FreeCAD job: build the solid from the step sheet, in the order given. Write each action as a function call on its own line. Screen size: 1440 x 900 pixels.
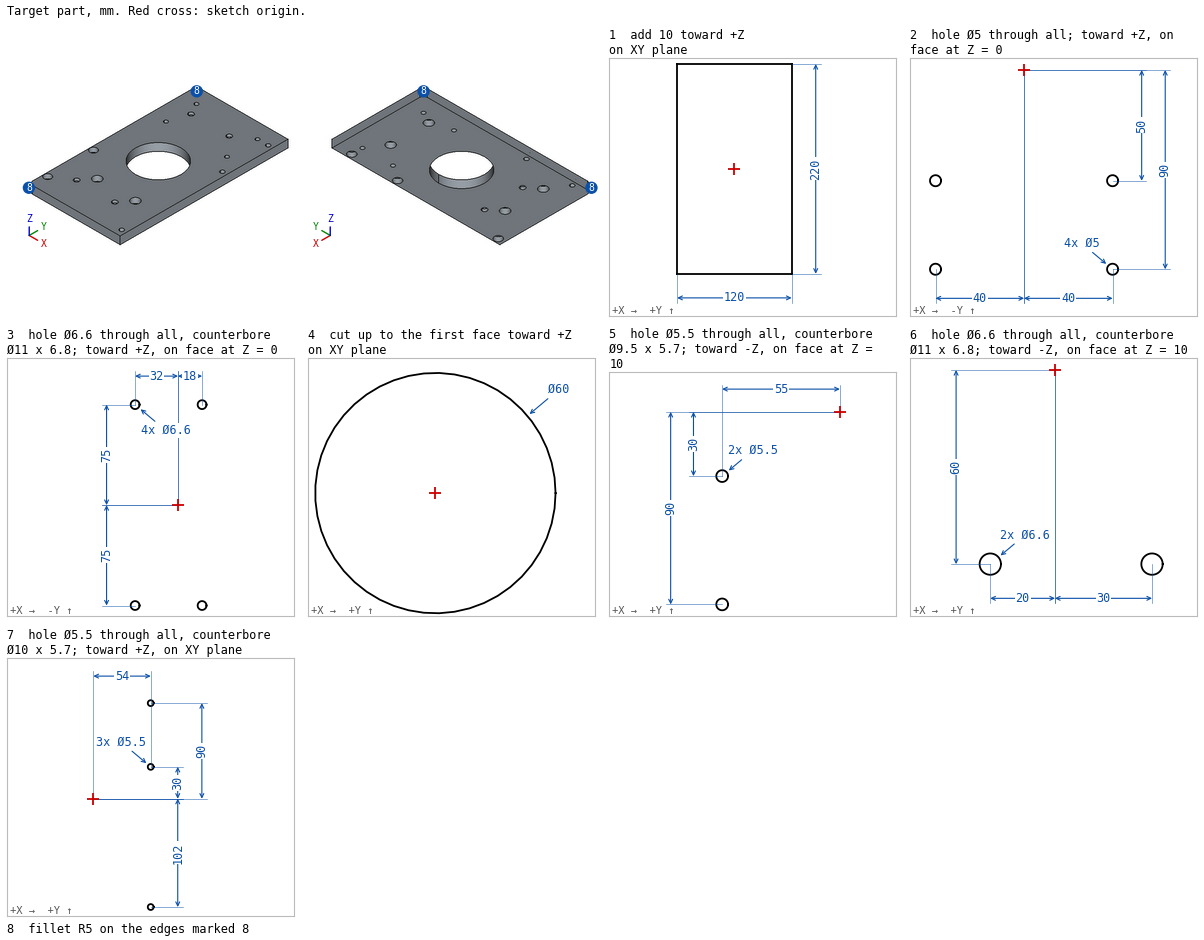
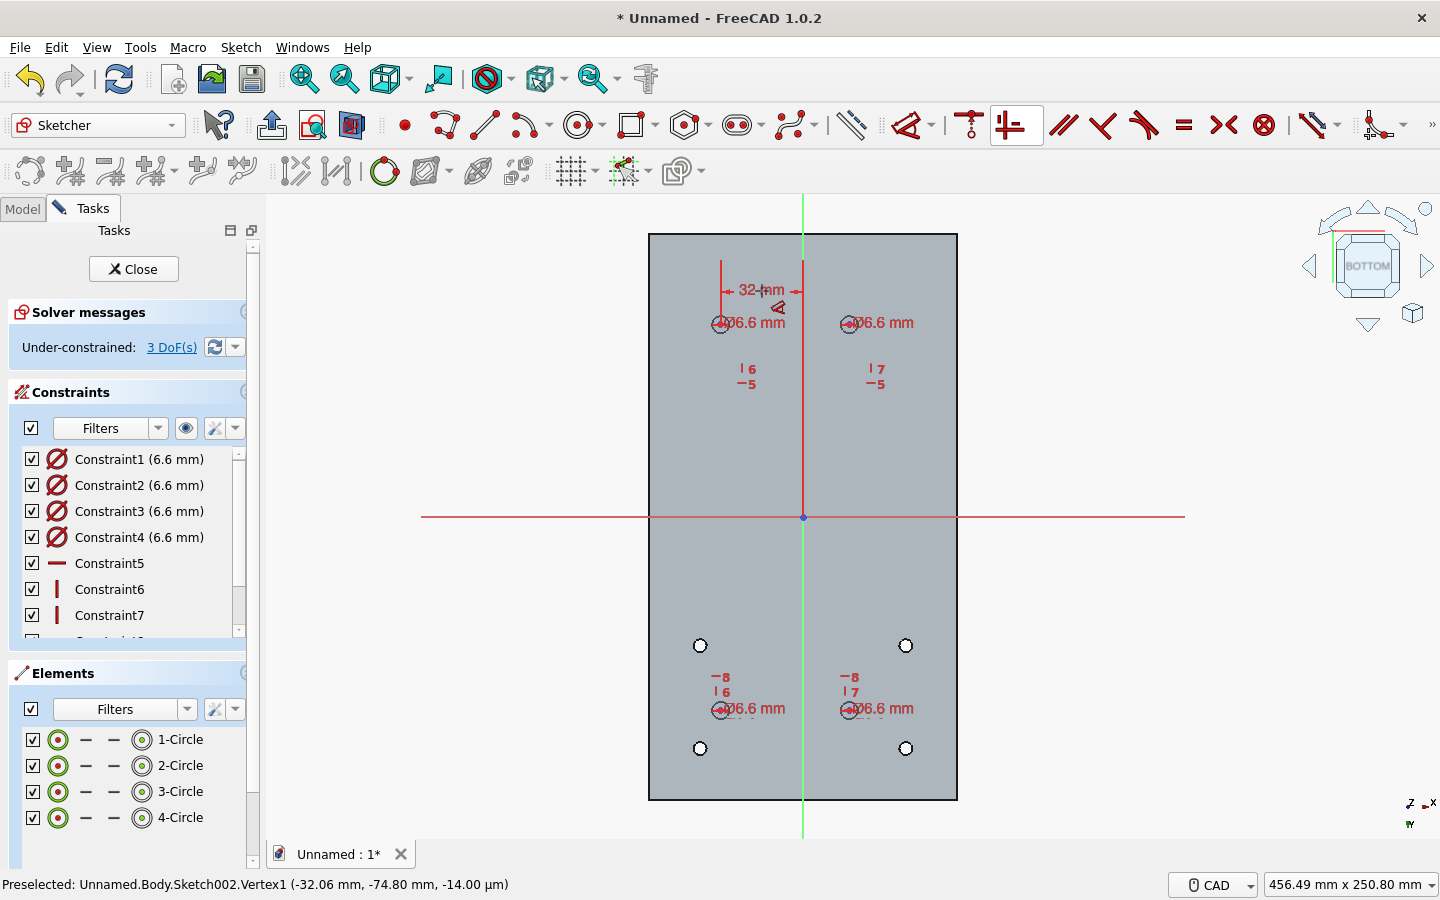
click(721, 325)
click(687, 421)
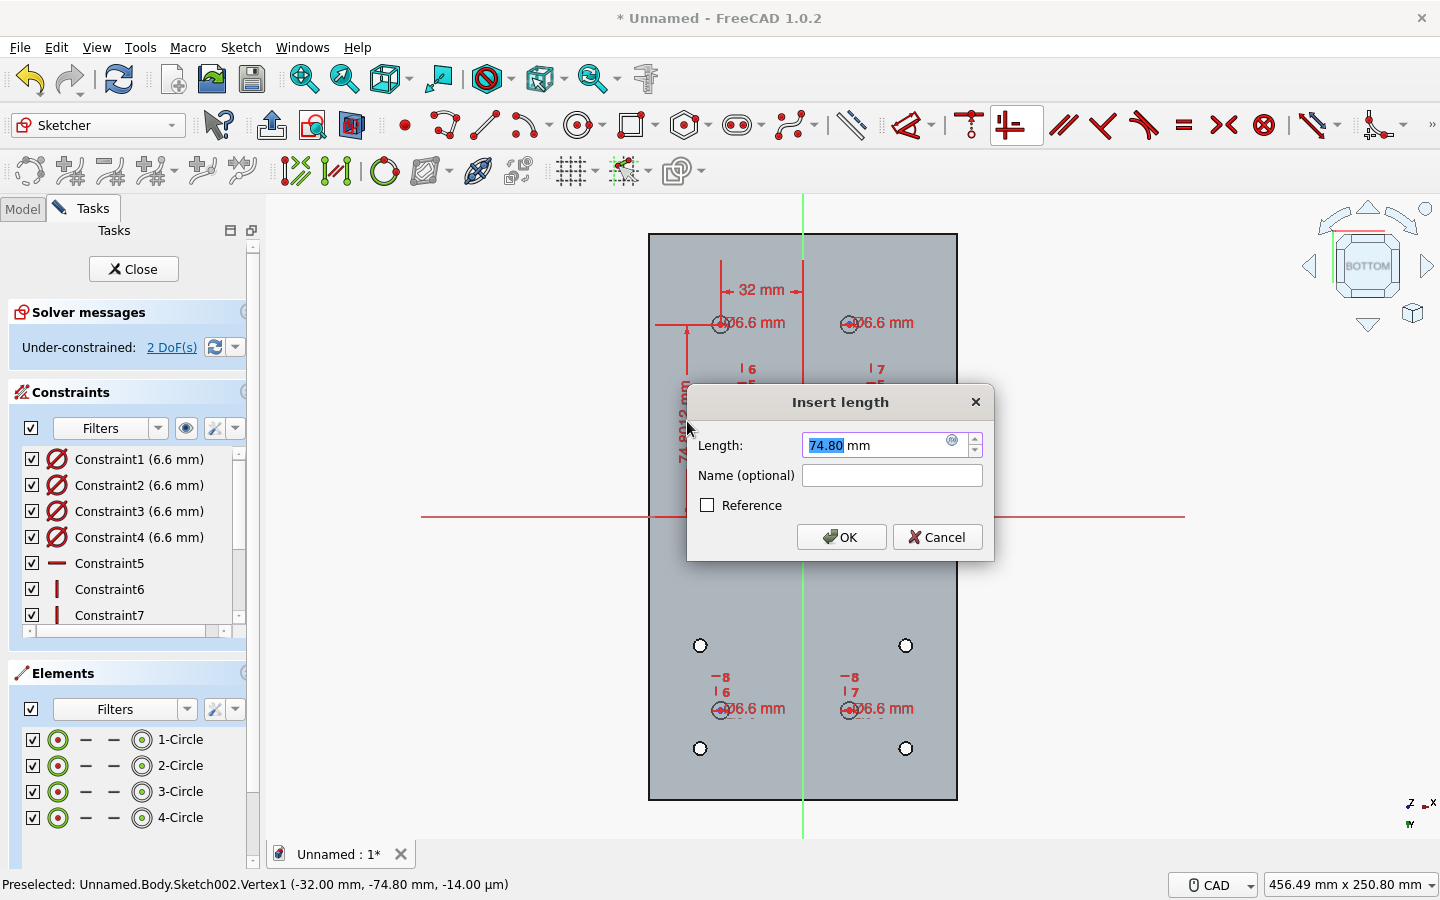
text(75)
key(Return)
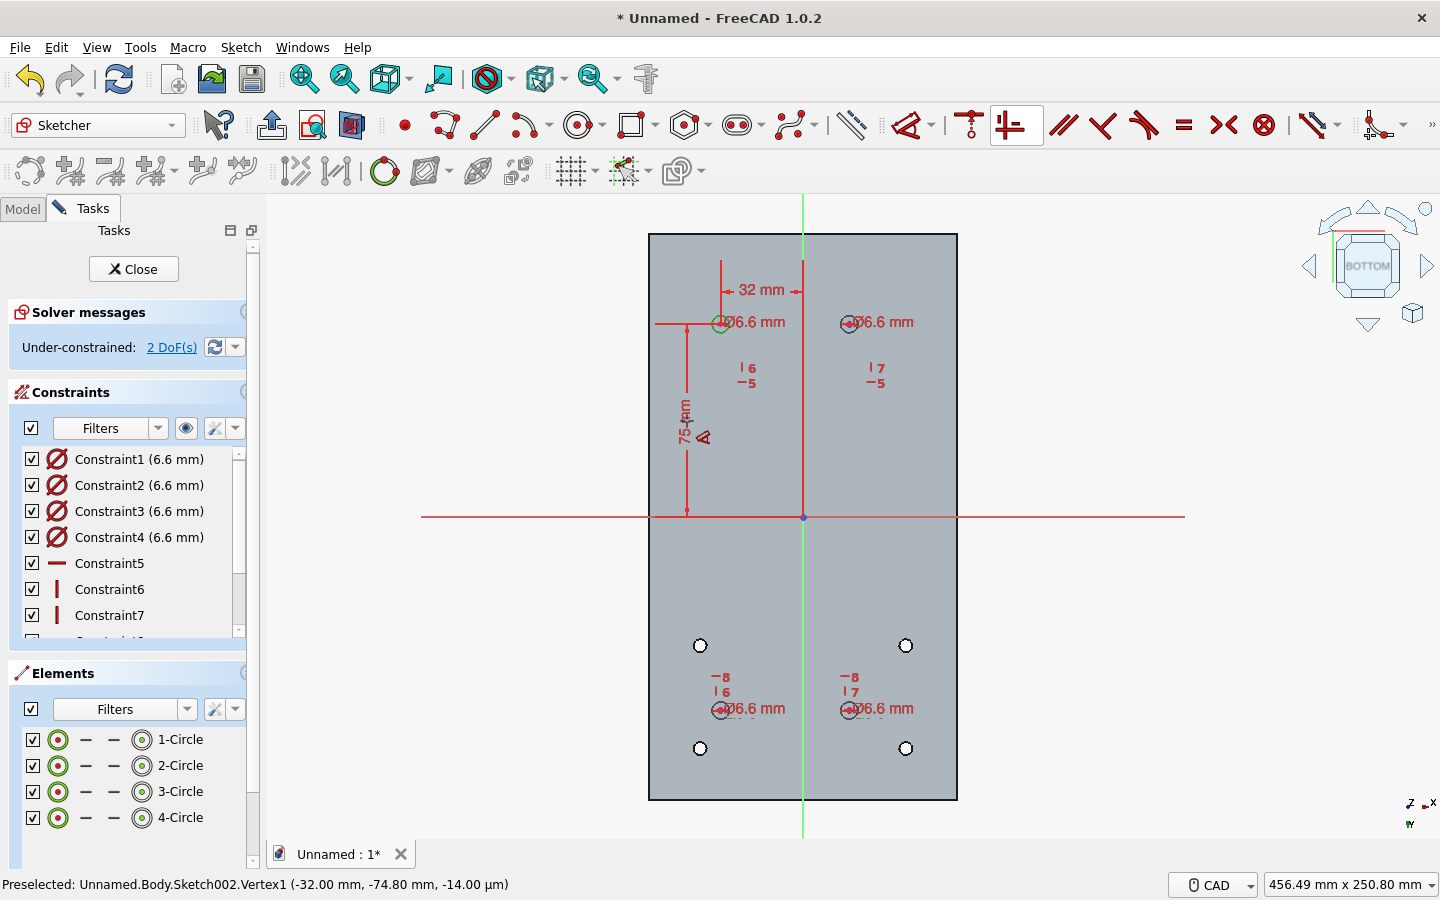
click(849, 324)
click(837, 290)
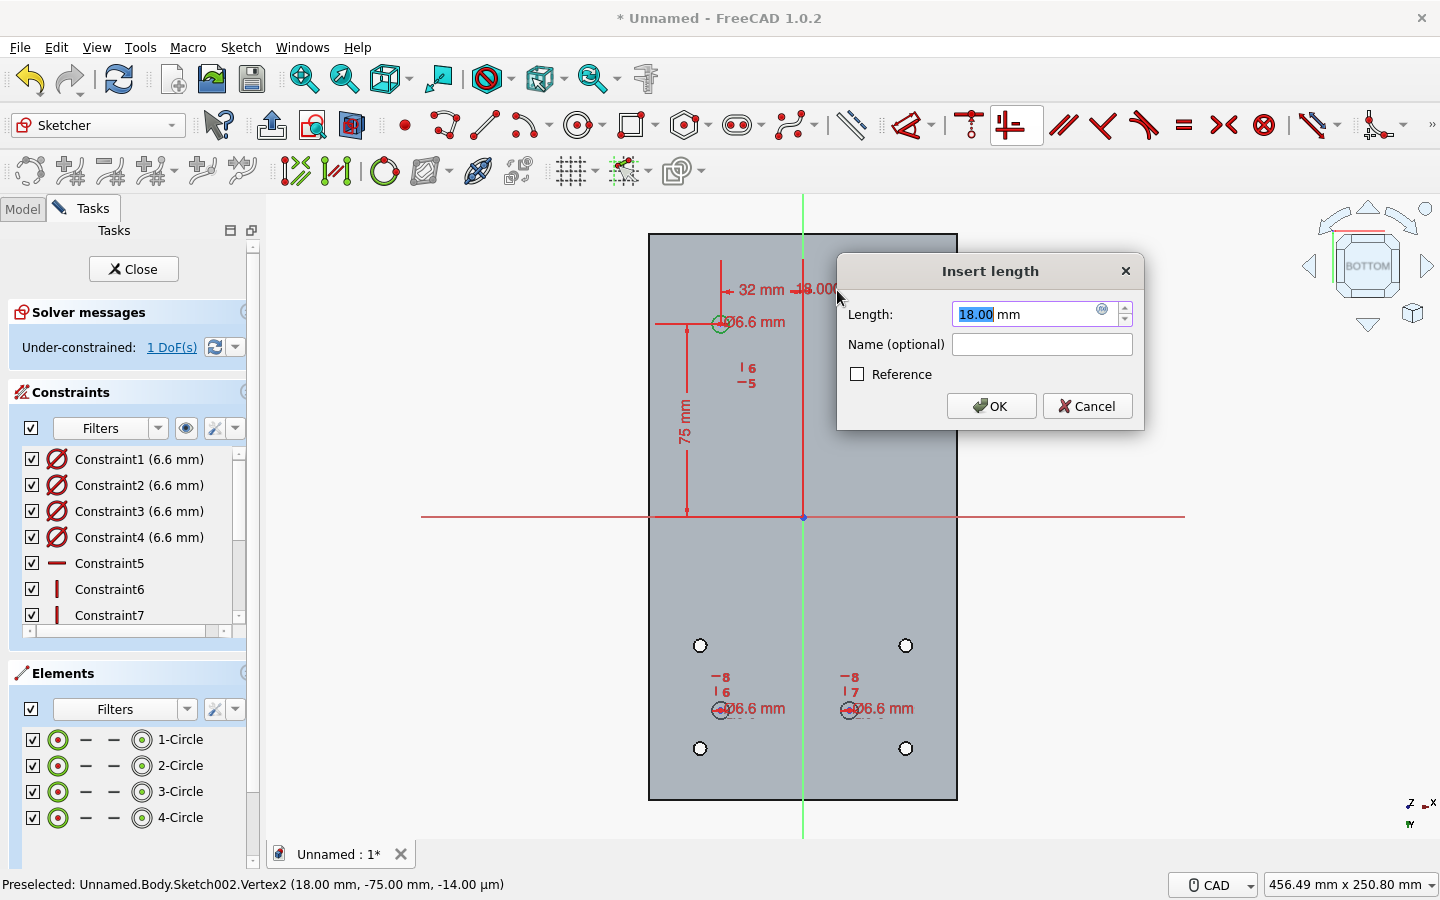
text(18)
key(Return)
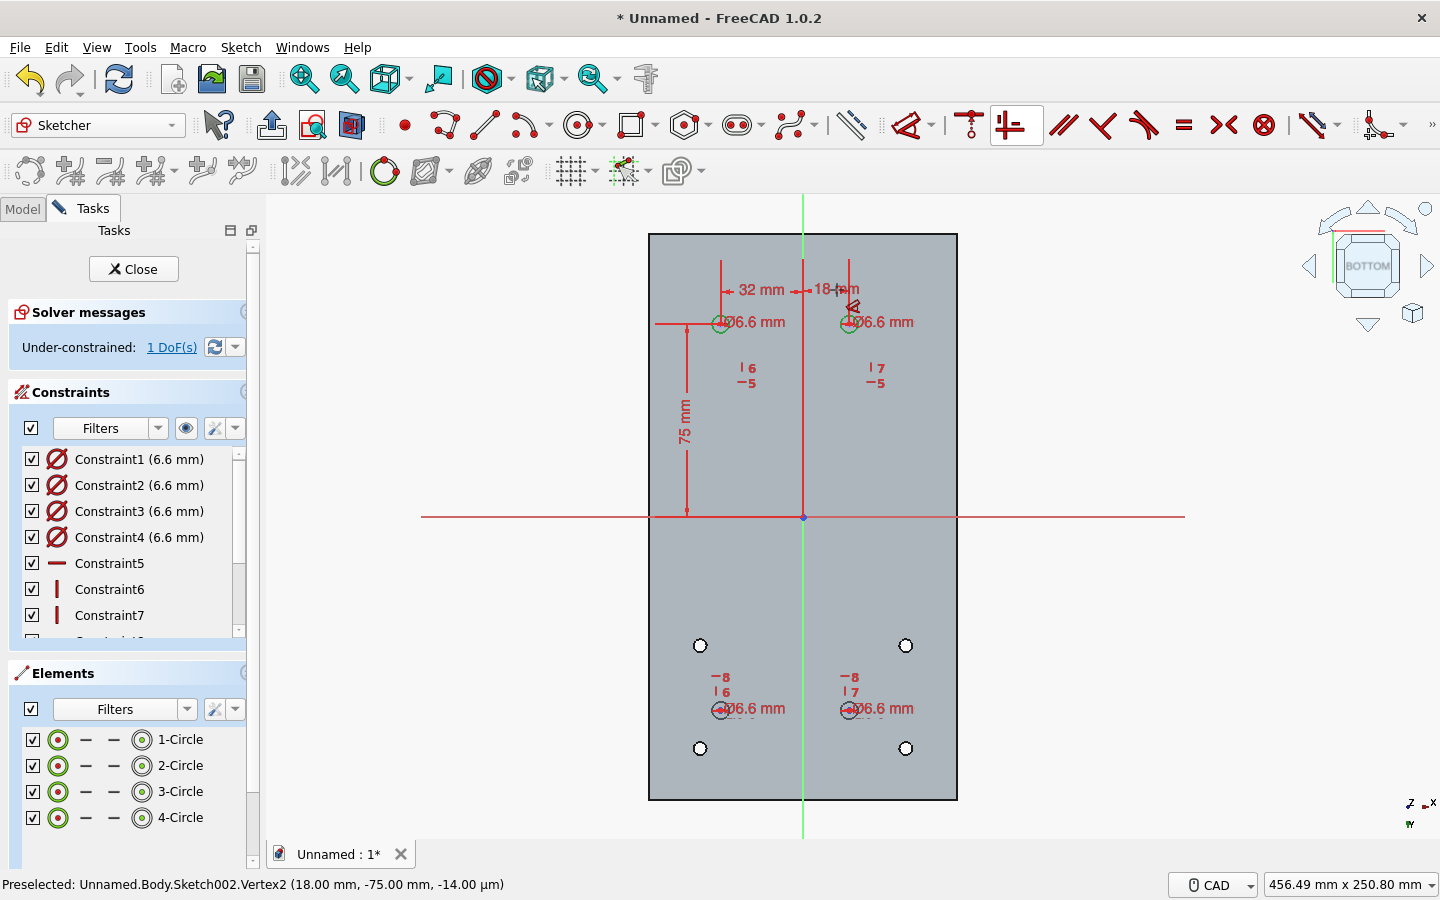
click(721, 711)
click(687, 614)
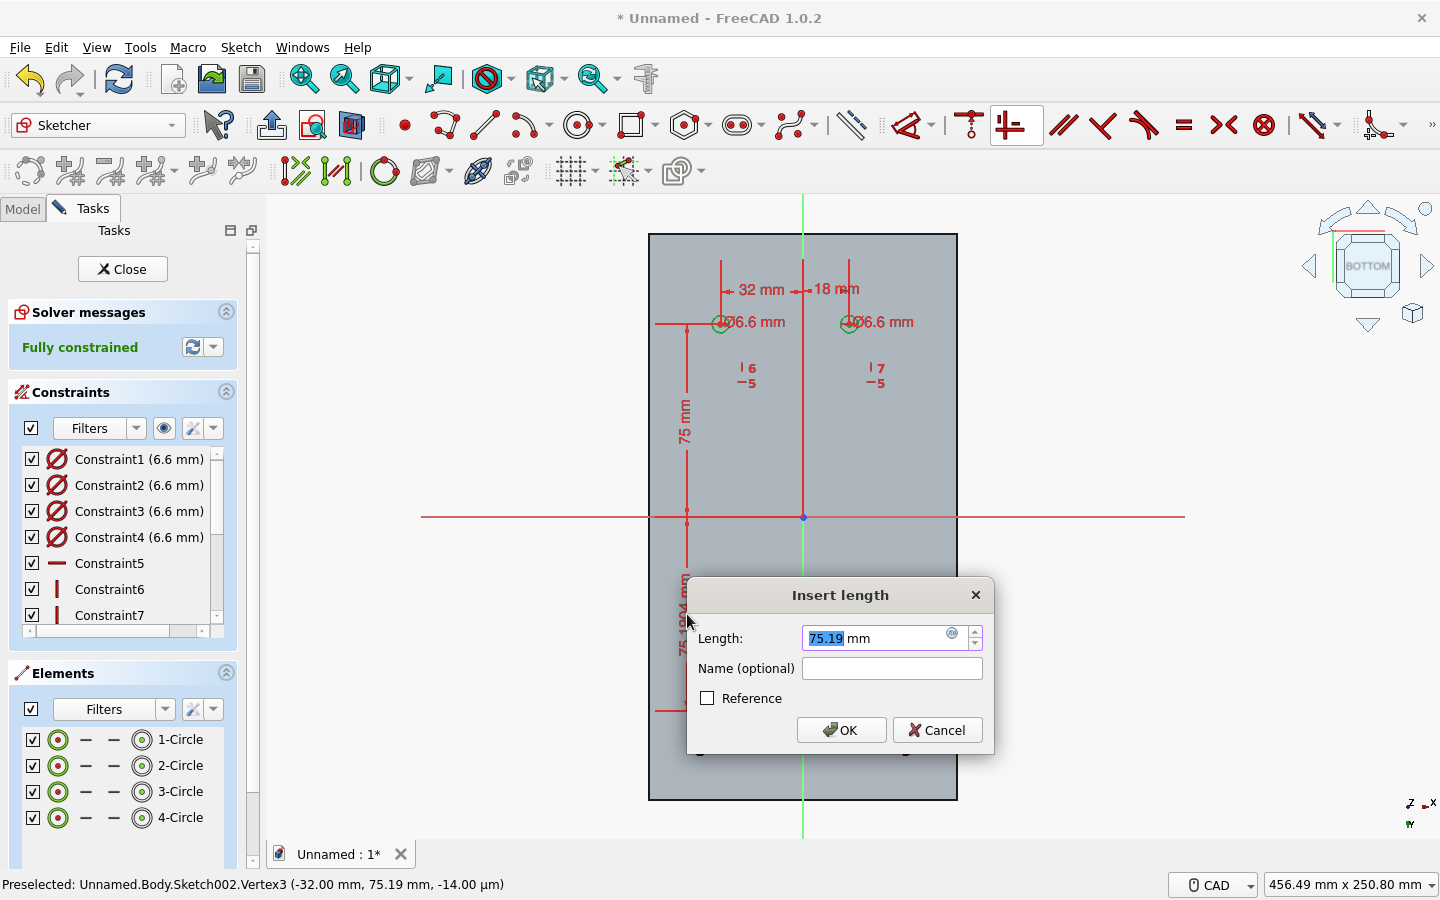
text(75)
key(Return)
key(Escape)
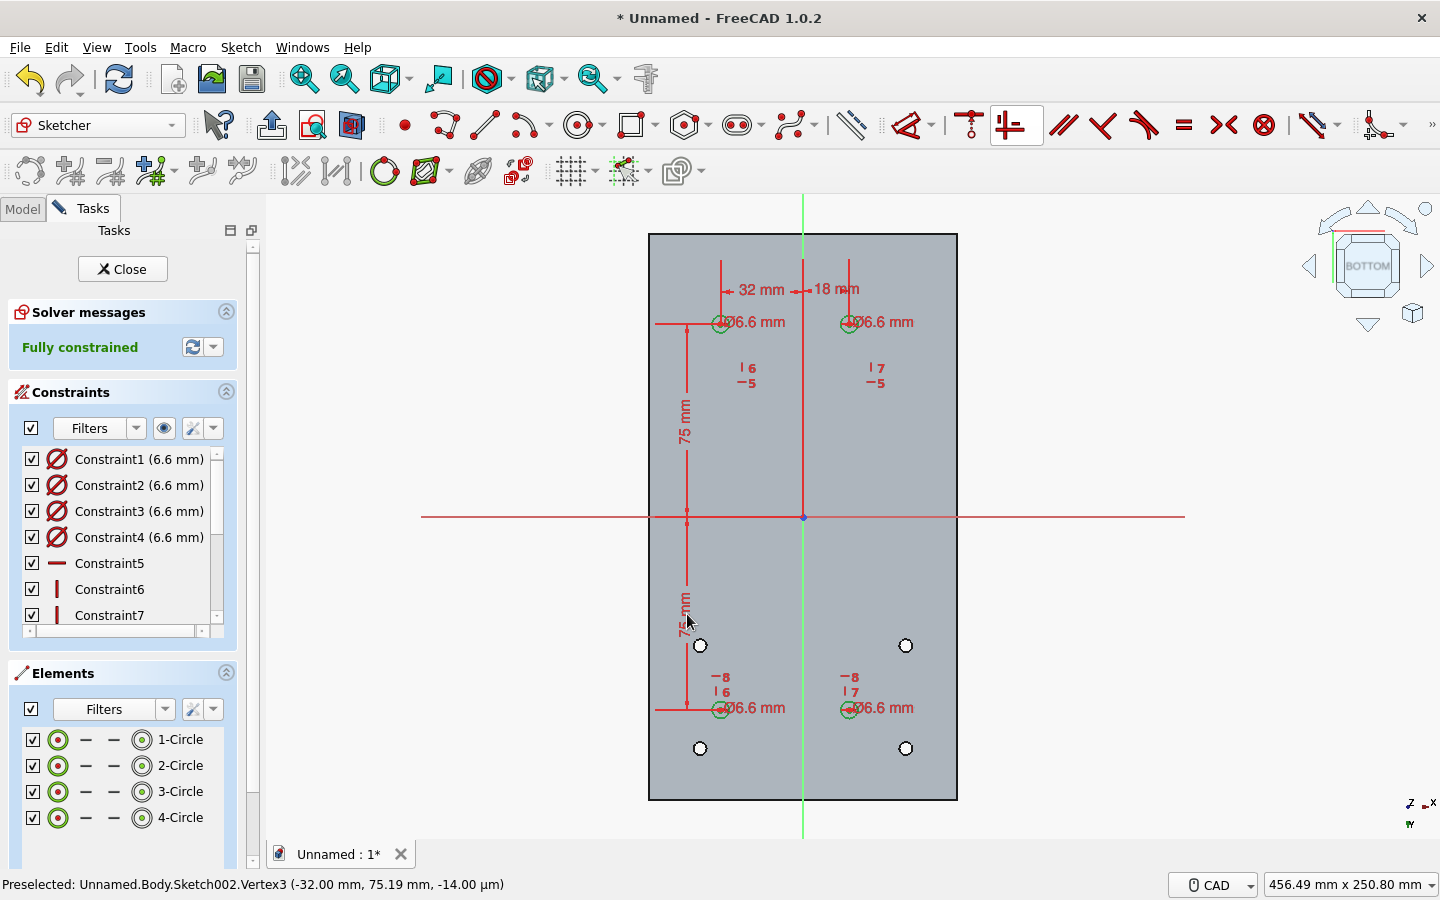
click(123, 269)